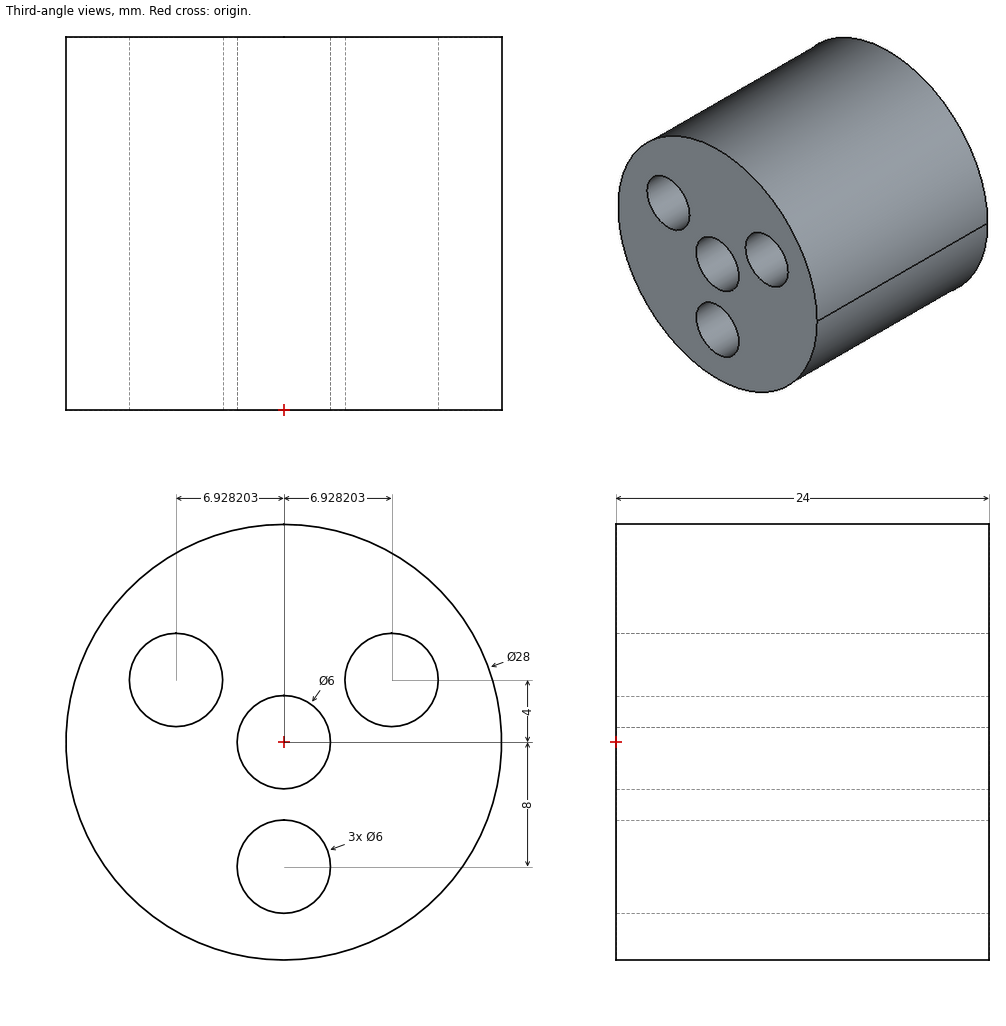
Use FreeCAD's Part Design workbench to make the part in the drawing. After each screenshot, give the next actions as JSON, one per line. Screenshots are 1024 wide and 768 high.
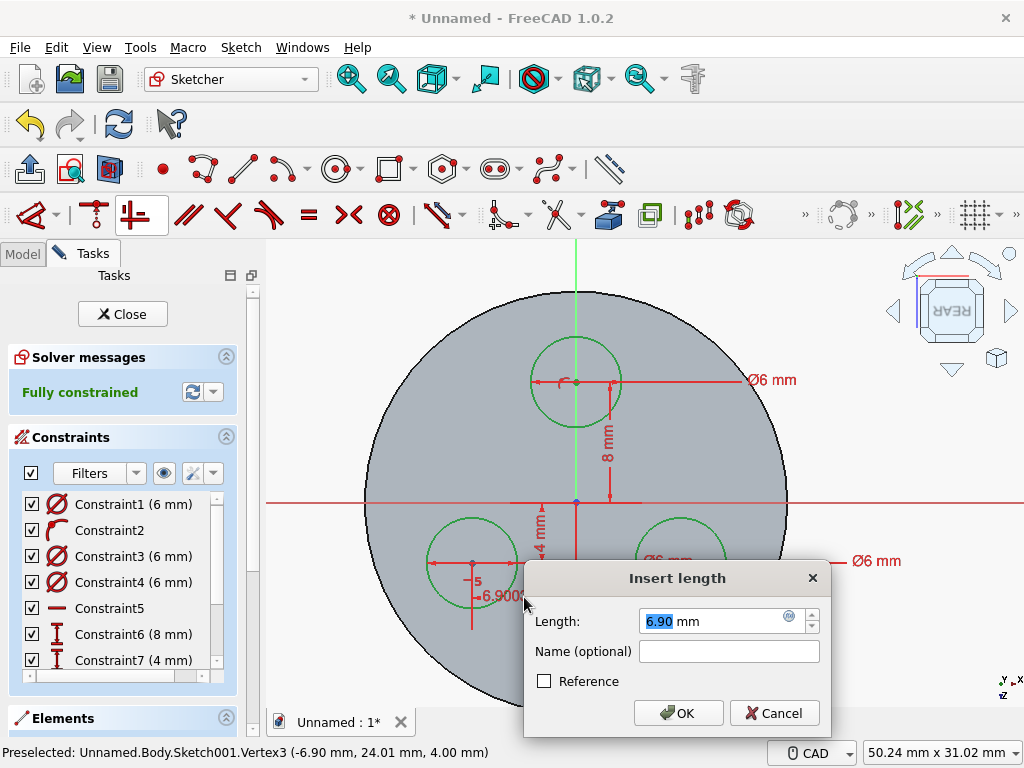
{"action": "type", "text": "6.928203"}
{"action": "key", "text": "Return"}
{"action": "key", "text": "Escape"}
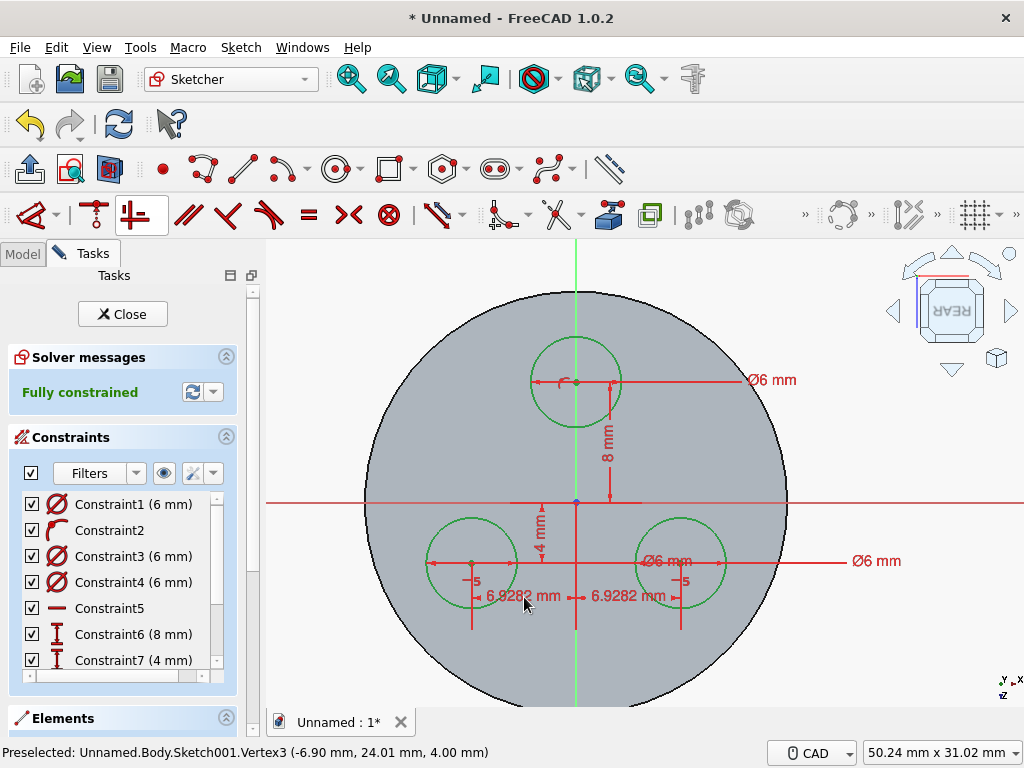
{"action": "left_click", "coordinate": [123, 314]}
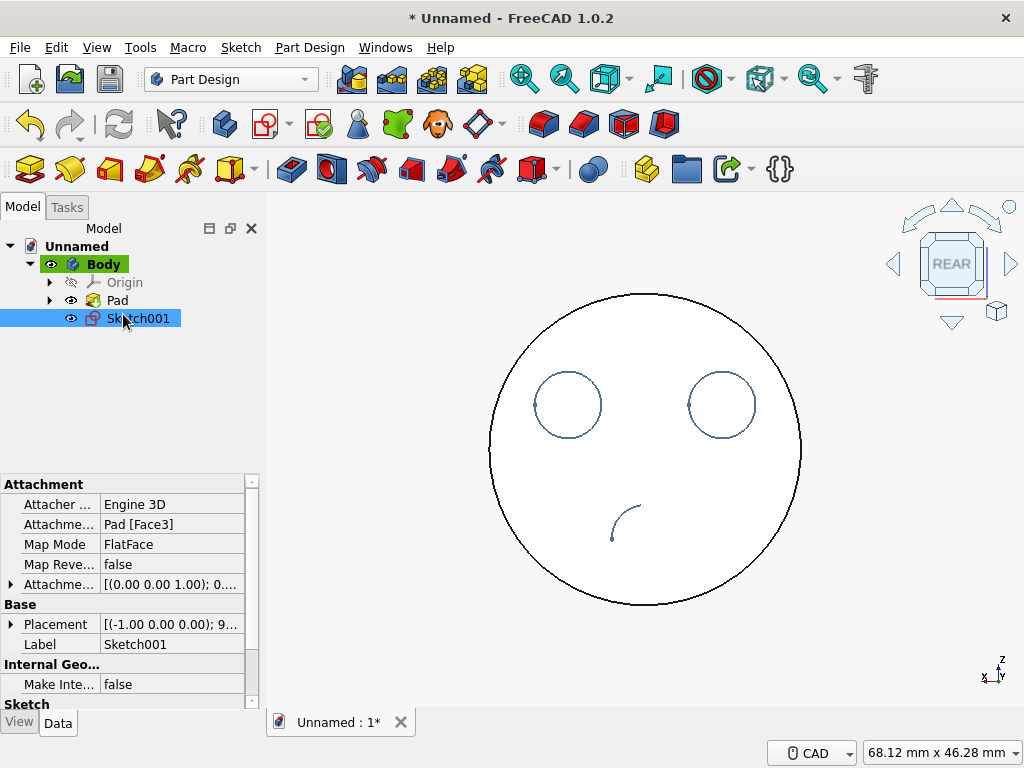
{"action": "left_click", "coordinate": [292, 170]}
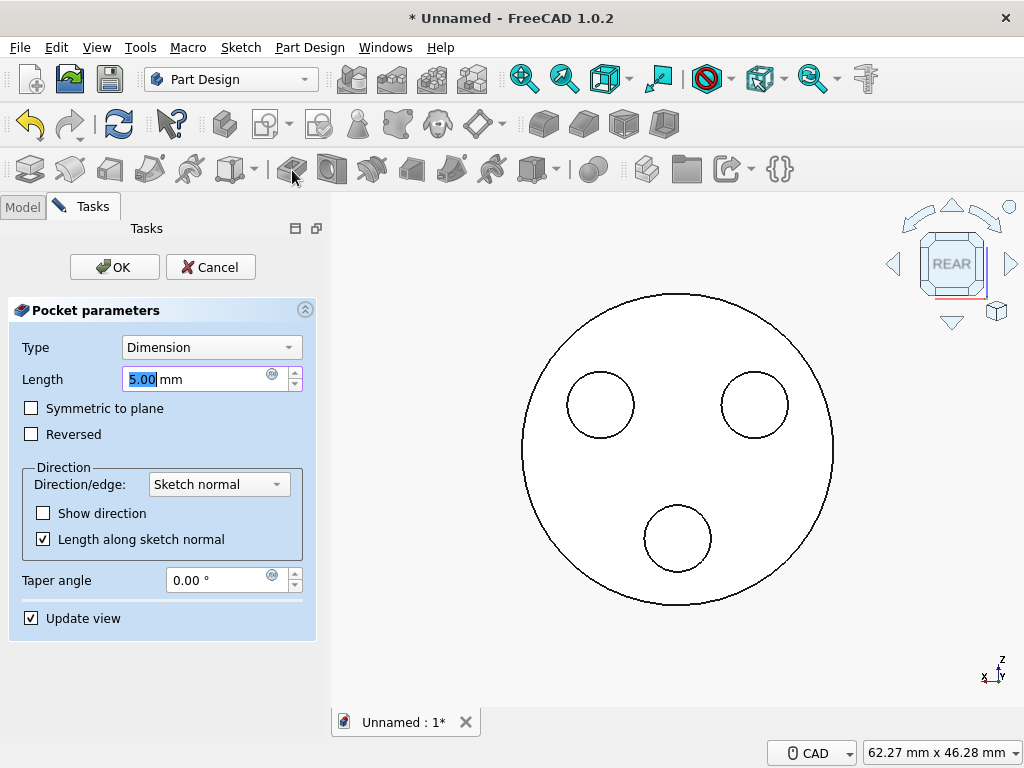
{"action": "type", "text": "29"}
{"action": "key", "text": "Tab"}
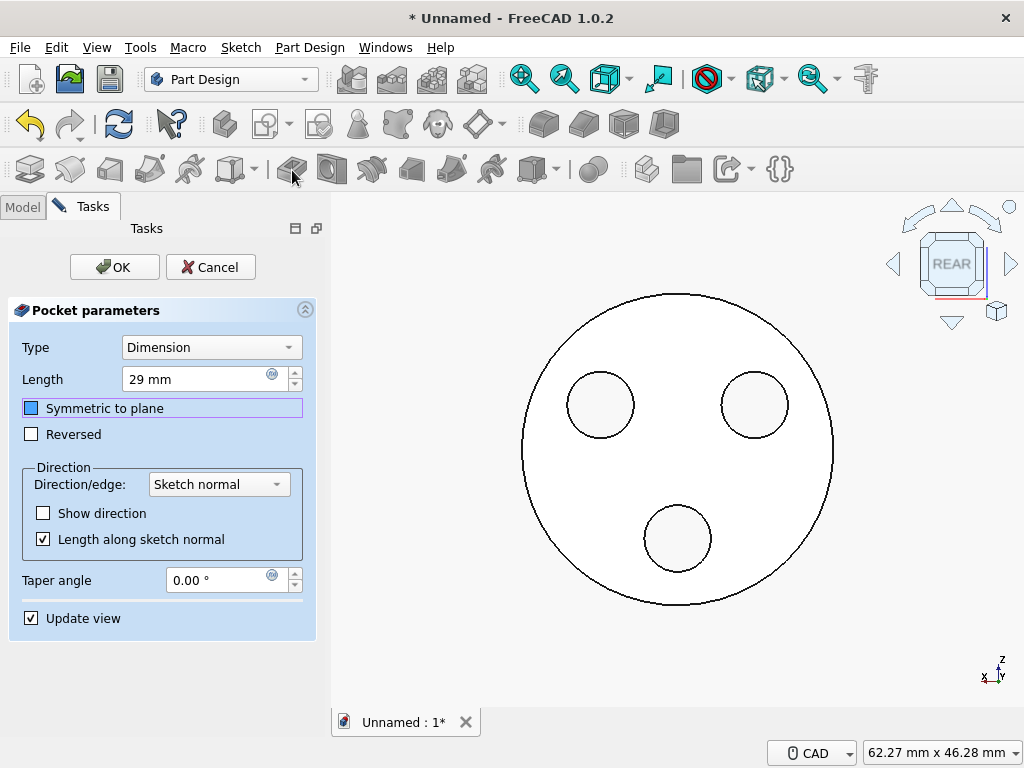
{"action": "left_click", "coordinate": [115, 267]}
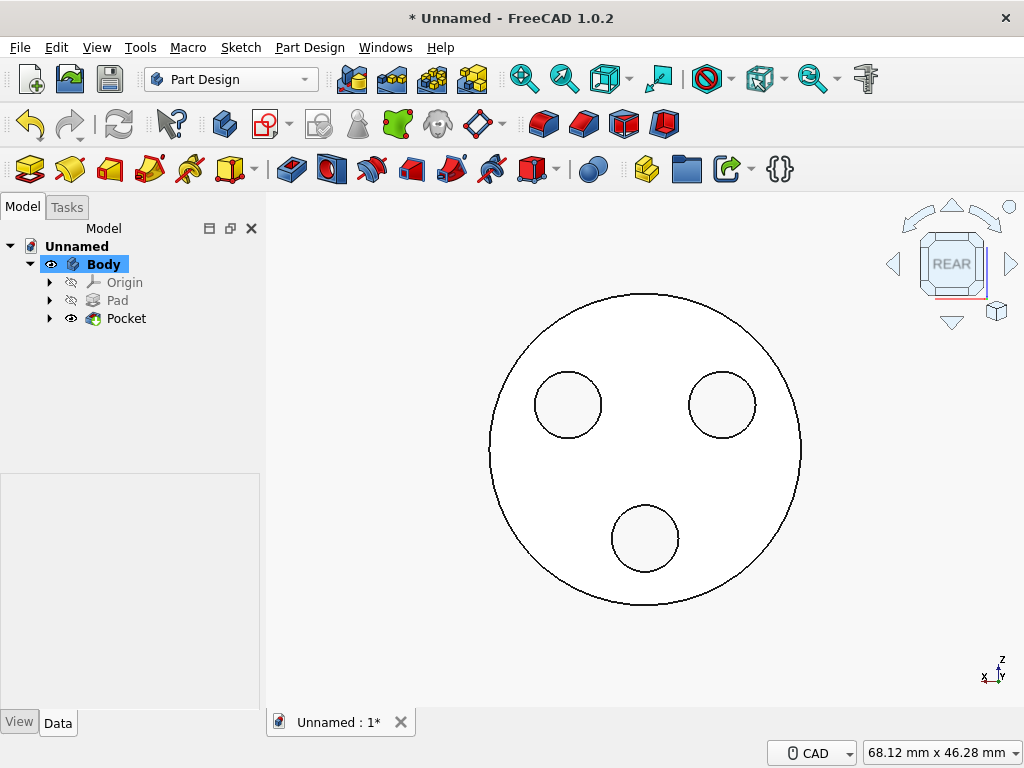
{"action": "left_click", "coordinate": [556, 493]}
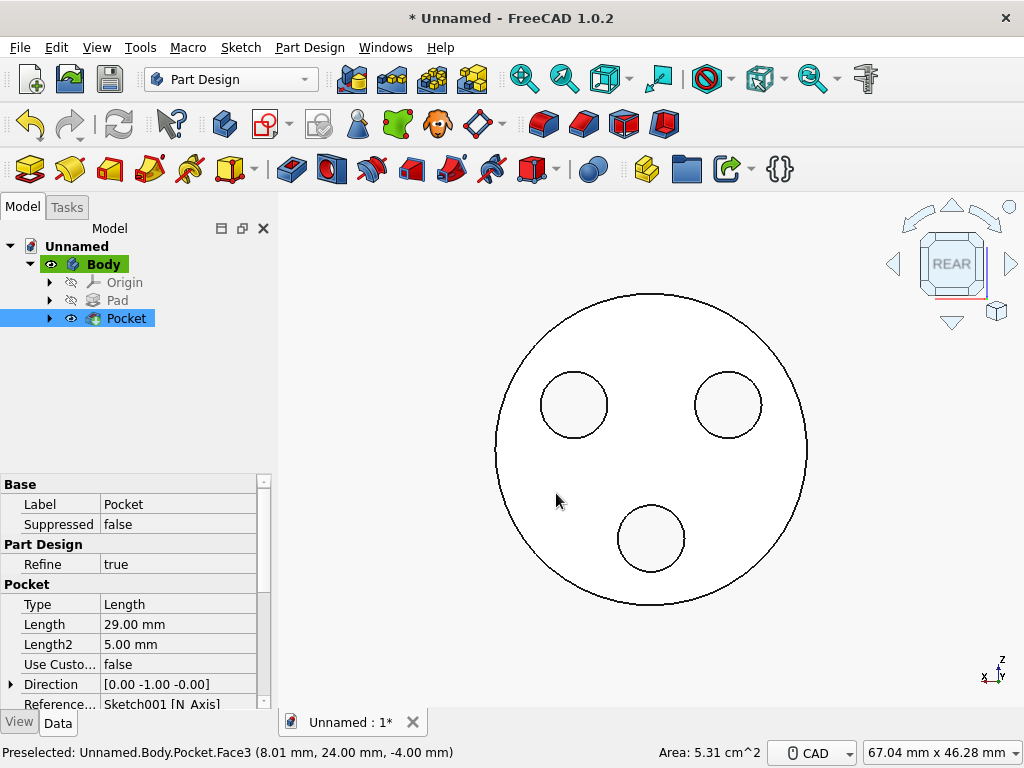
{"action": "left_click", "coordinate": [266, 124]}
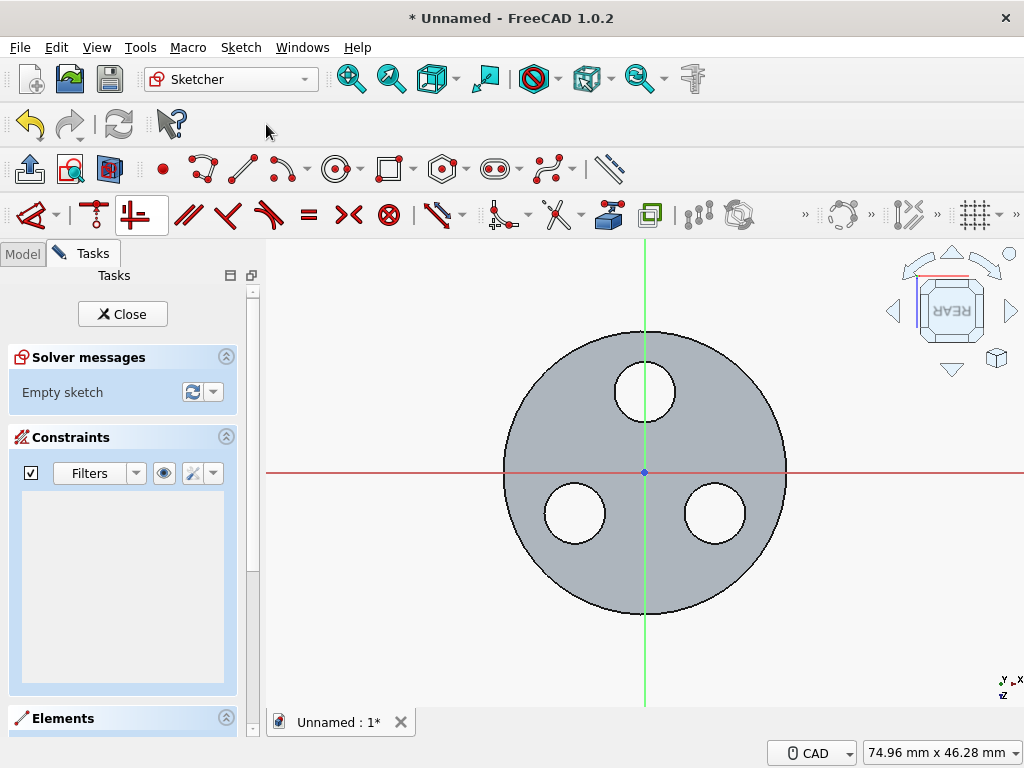
{"action": "scroll", "coordinate": [662, 473], "scroll_direction": "up", "scroll_amount": 8}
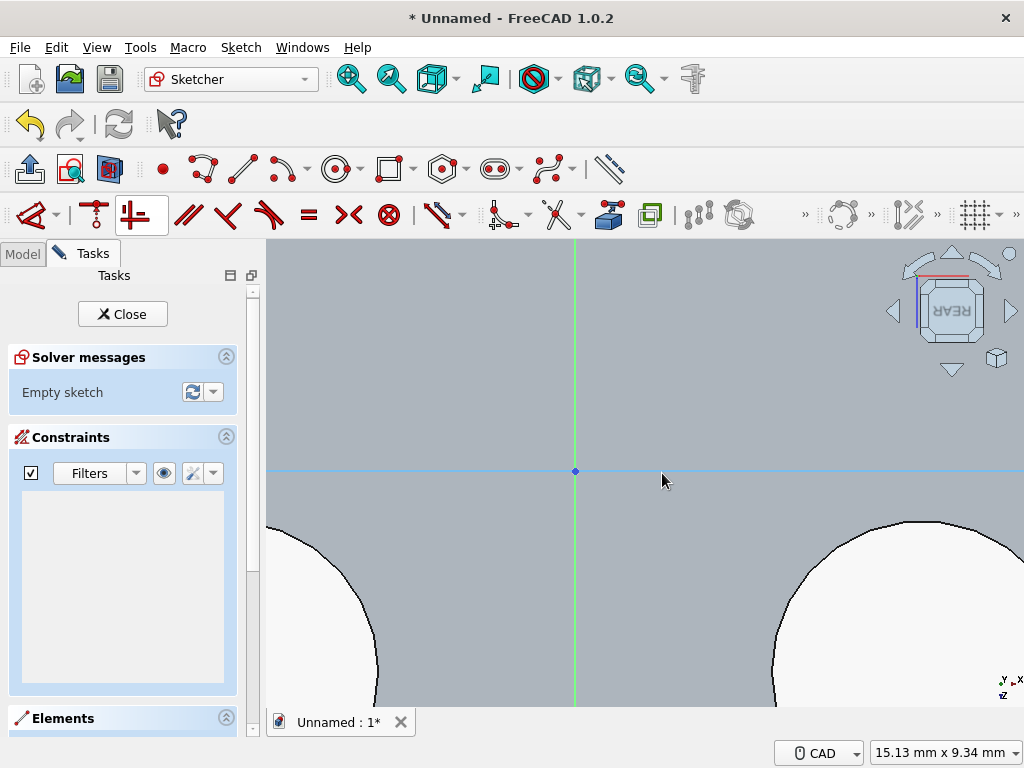
{"action": "left_click", "coordinate": [336, 170]}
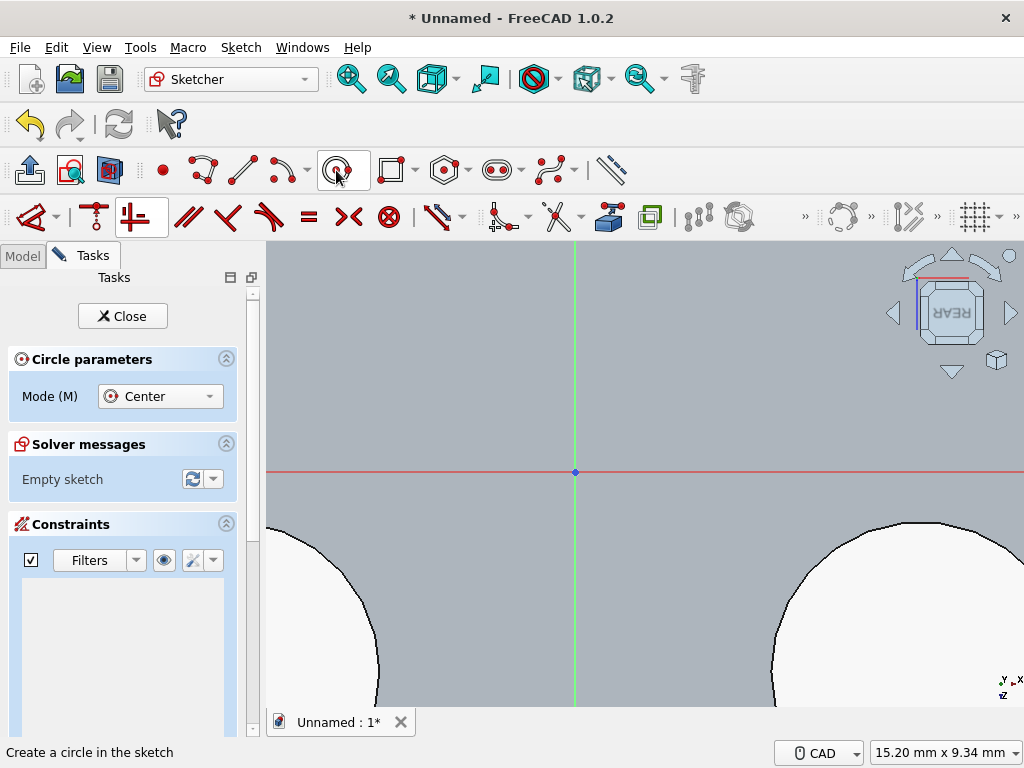
{"action": "left_click", "coordinate": [575, 472]}
{"action": "mouse_move", "coordinate": [681, 366]}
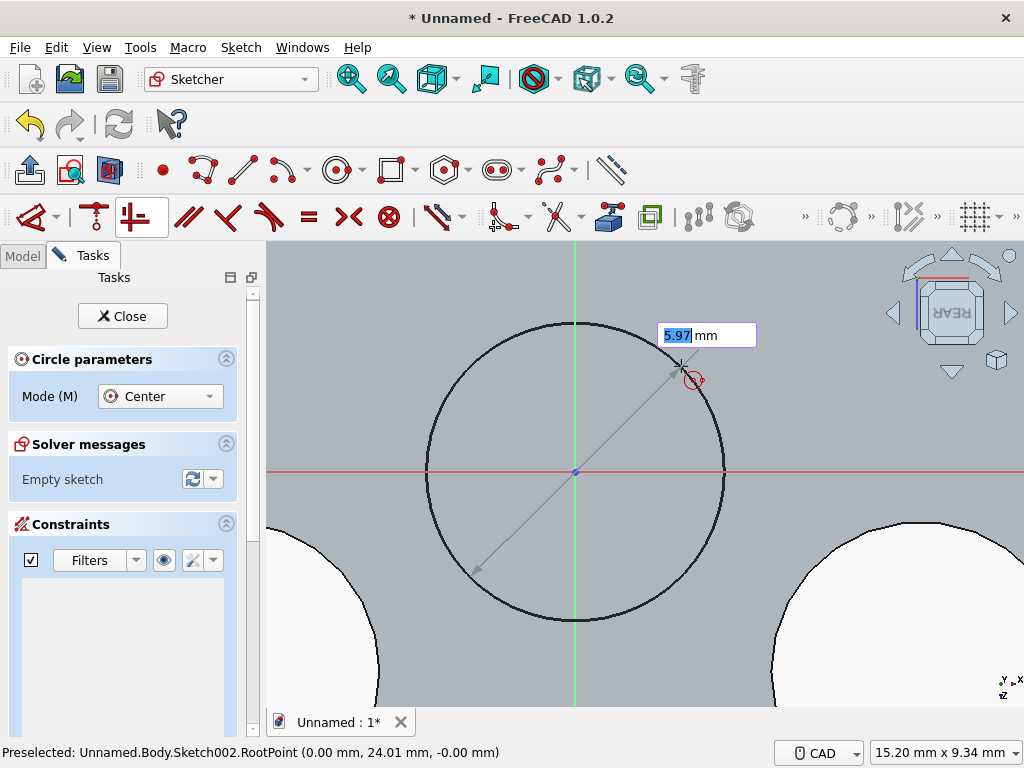
{"action": "type", "text": "6"}
{"action": "key", "text": "Return"}
{"action": "key", "text": "Escape"}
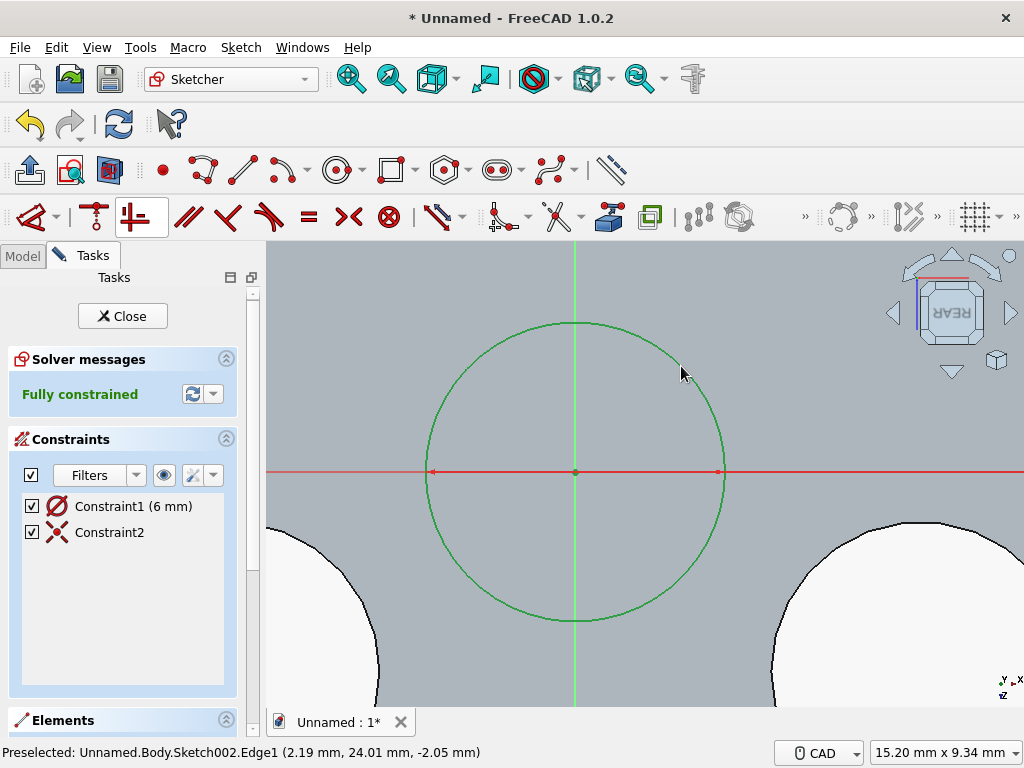
{"action": "left_click", "coordinate": [123, 316]}